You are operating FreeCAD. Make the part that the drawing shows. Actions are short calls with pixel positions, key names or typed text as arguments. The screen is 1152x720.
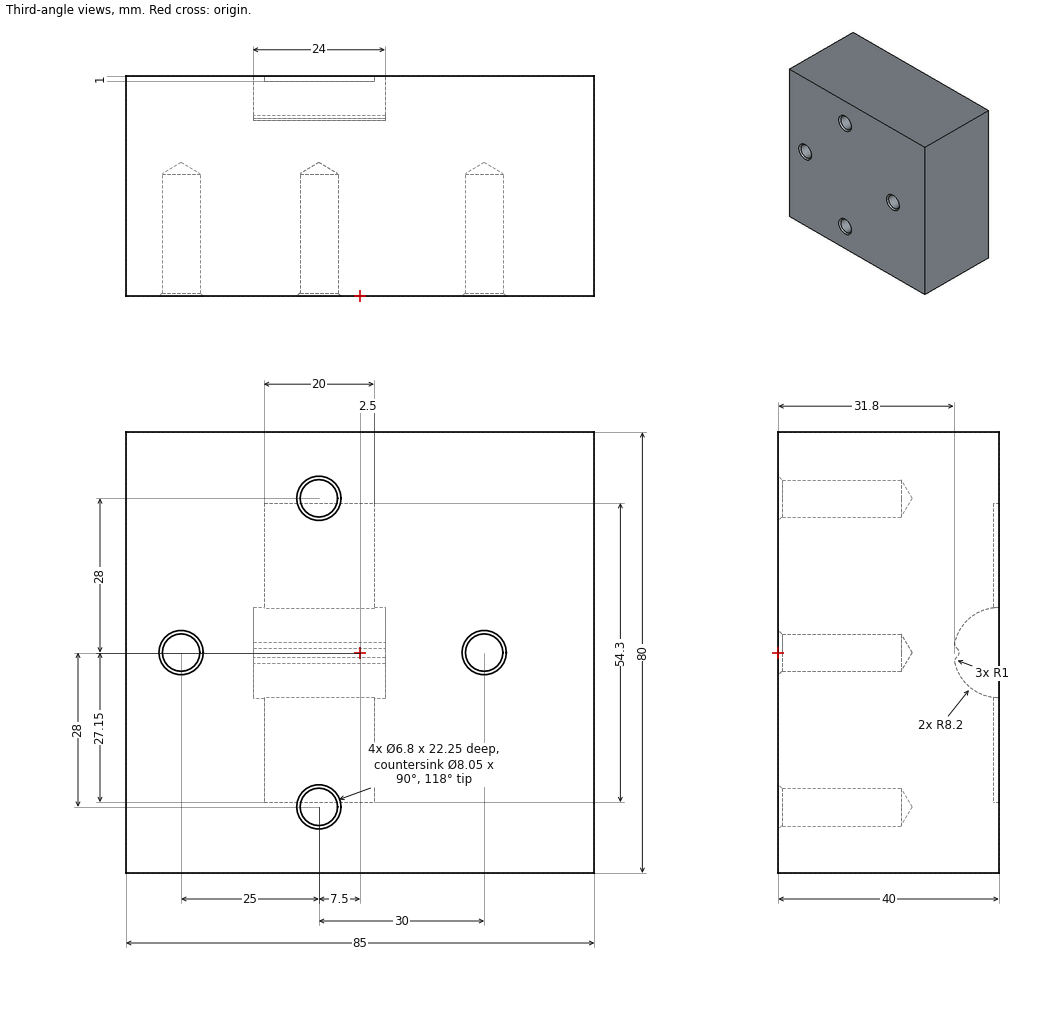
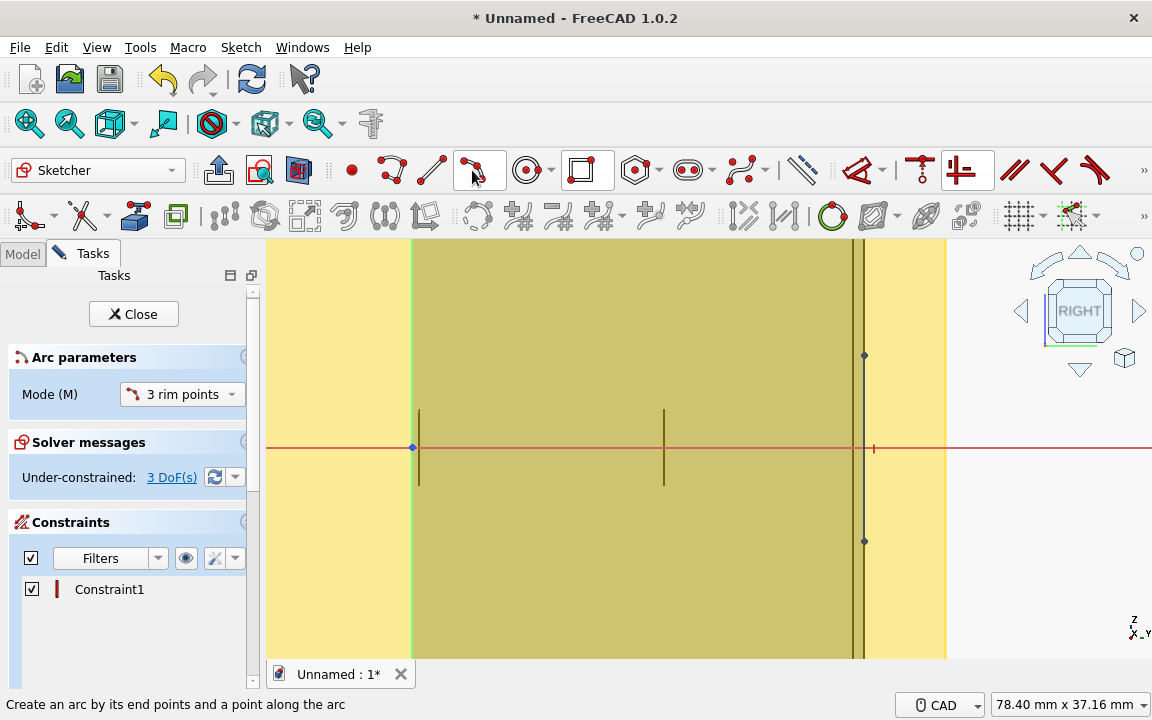
click(864, 542)
click(774, 469)
click(806, 520)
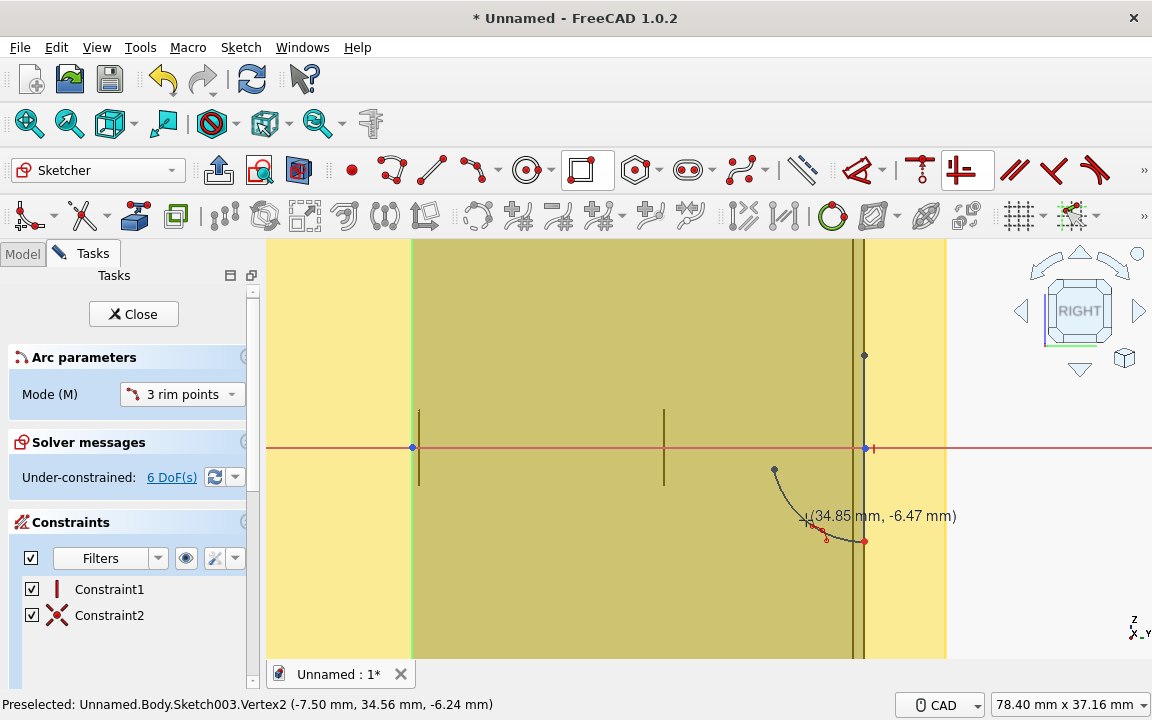
click(774, 470)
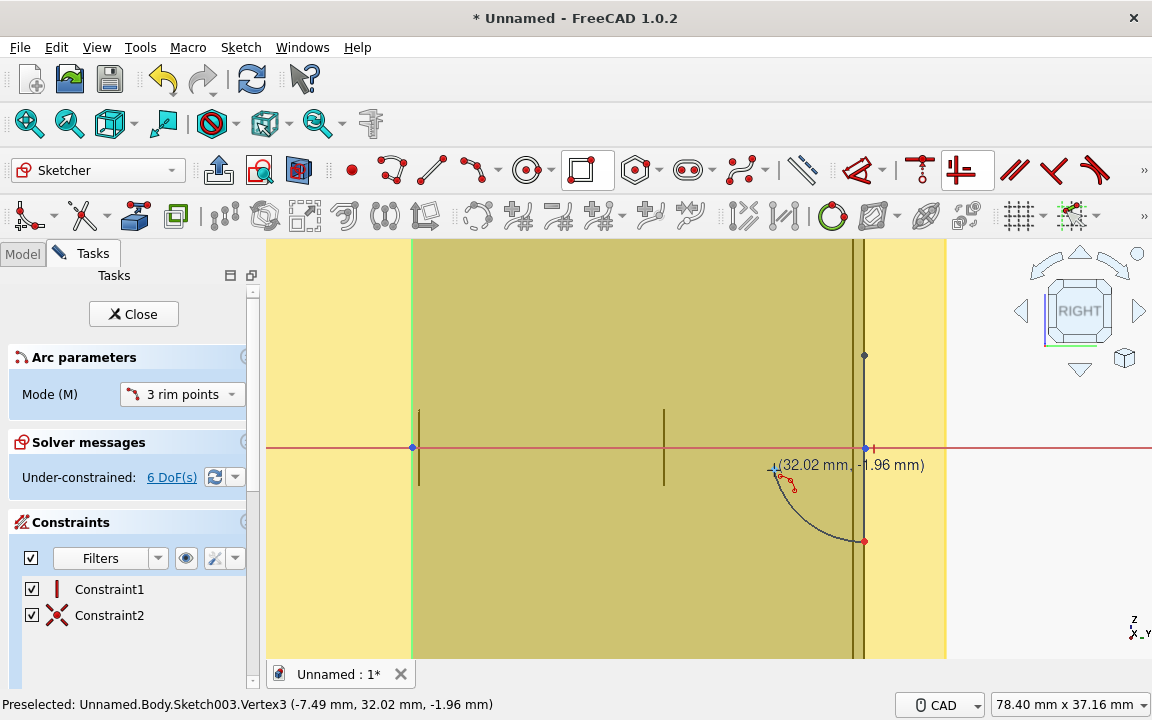
scroll(778, 457, up, 3)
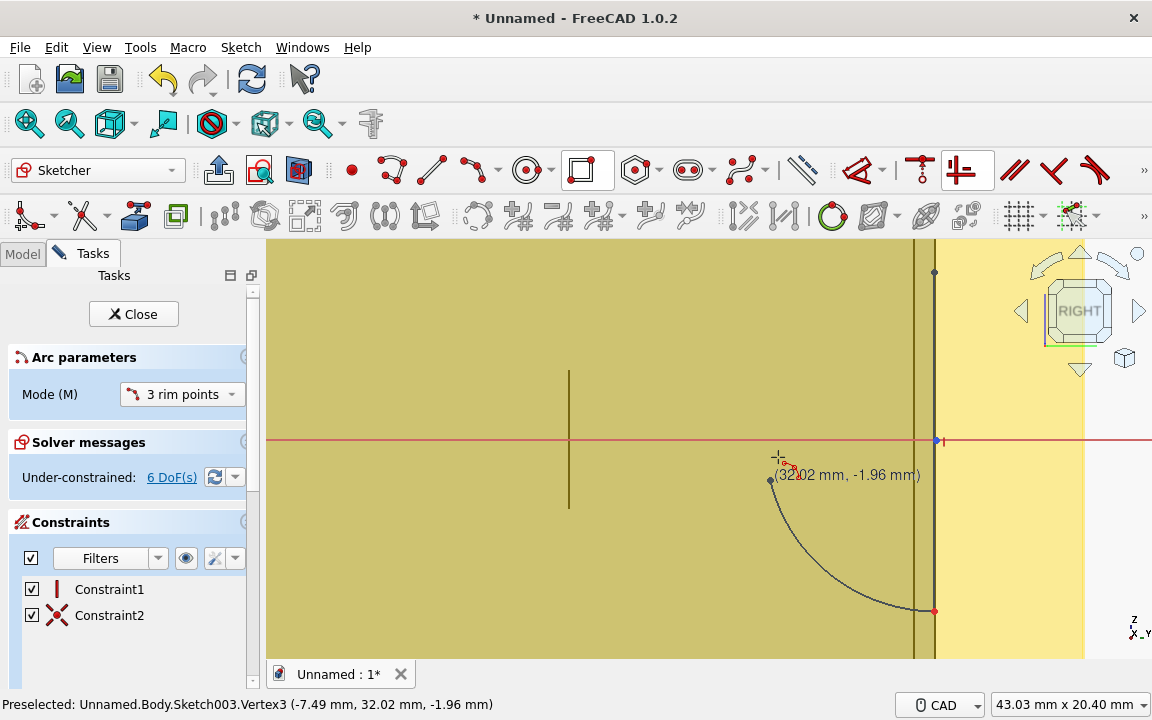
click(778, 456)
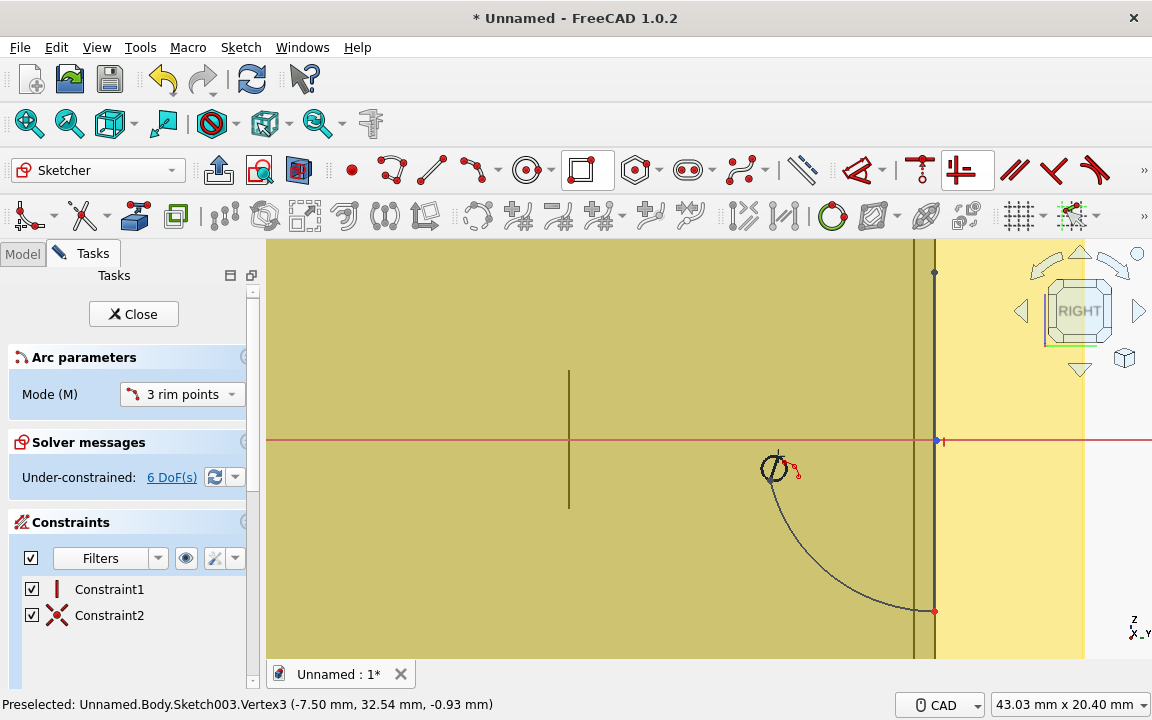
scroll(771, 466, up, 8)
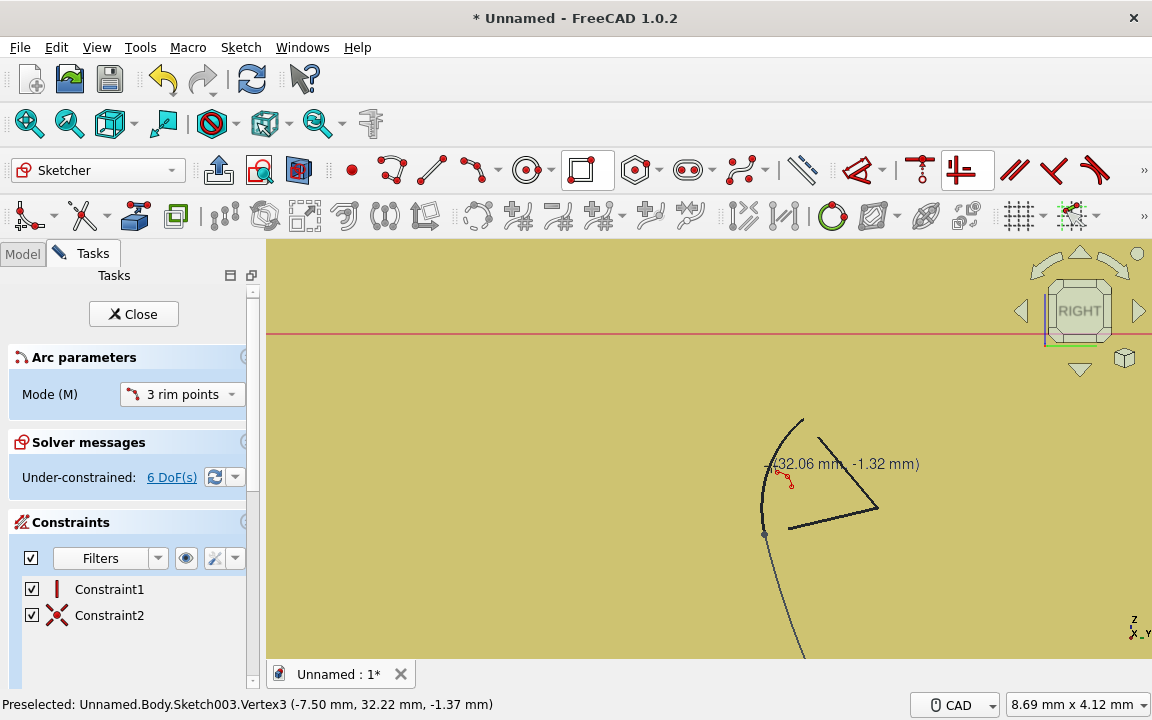
click(768, 463)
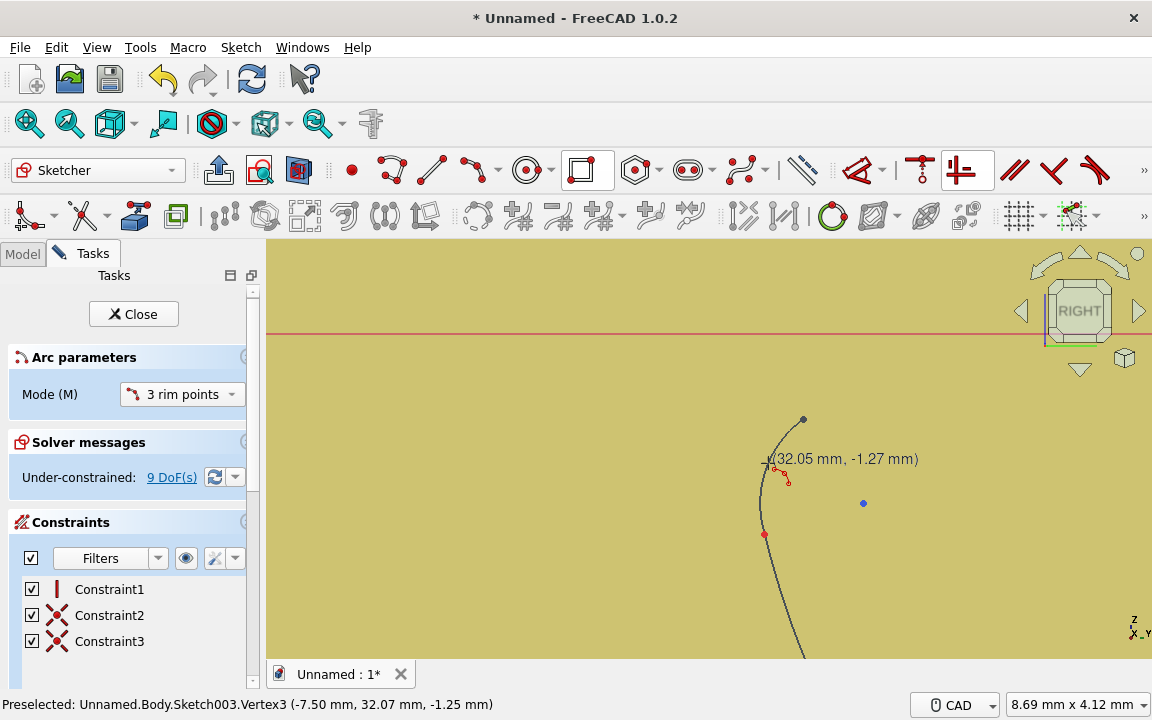
scroll(778, 463, down, 11)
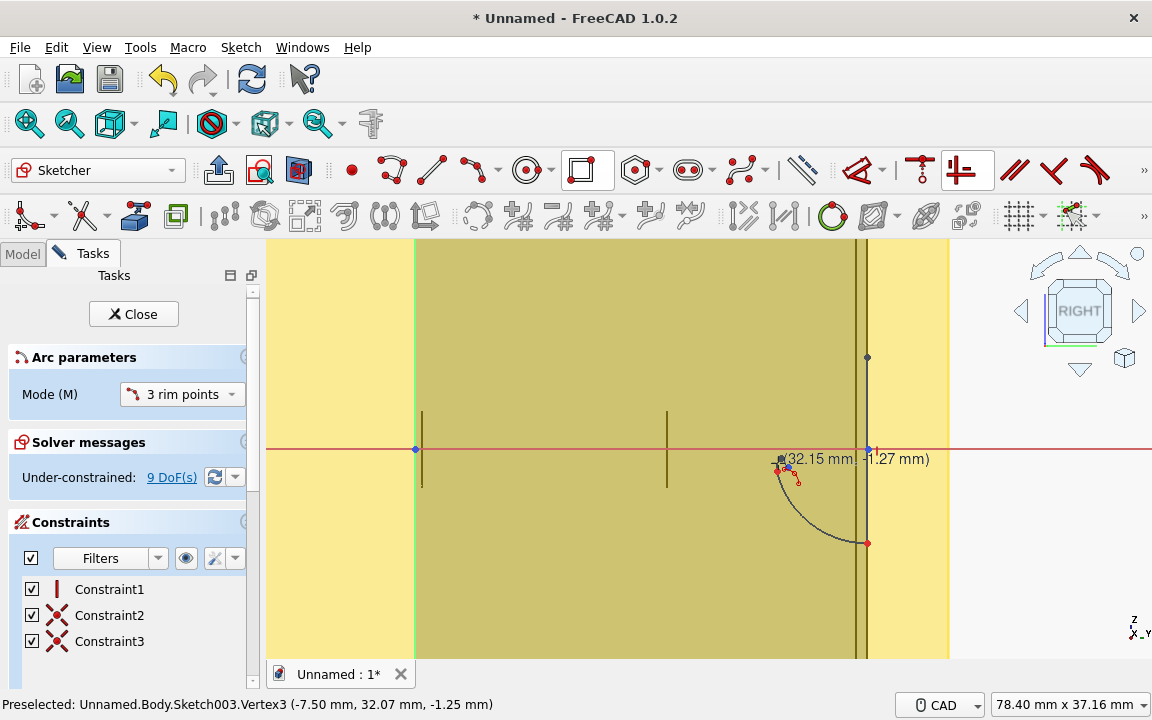
scroll(781, 458, up, 3)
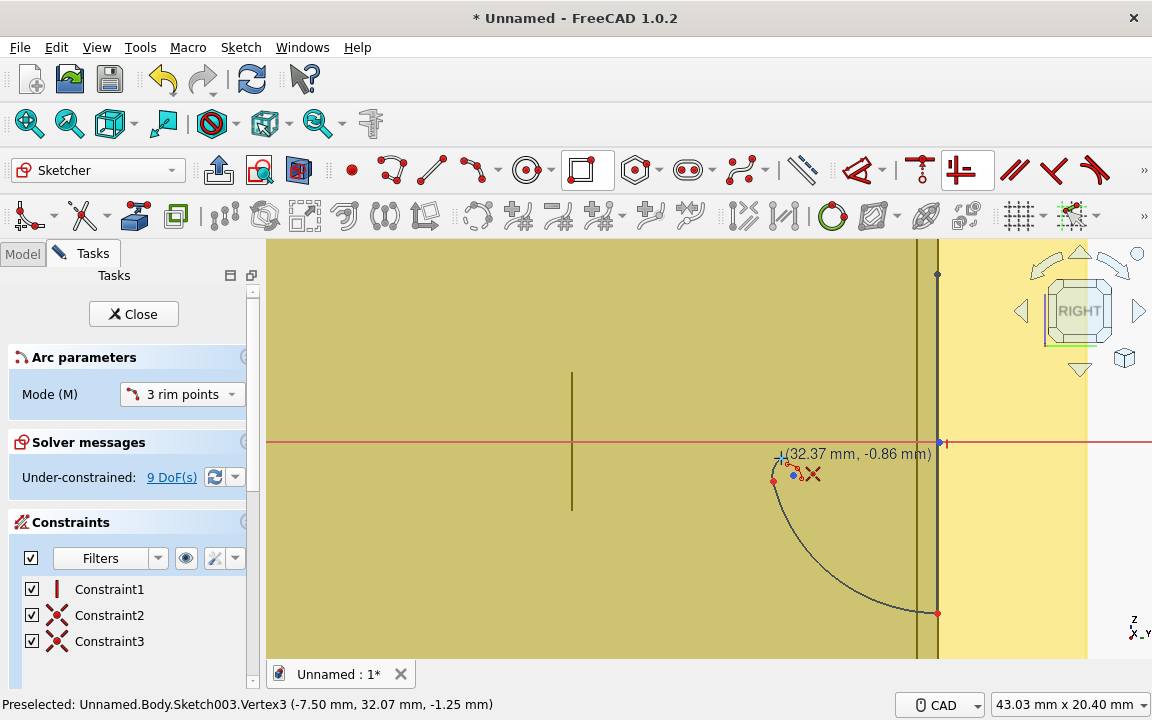
click(781, 459)
click(781, 425)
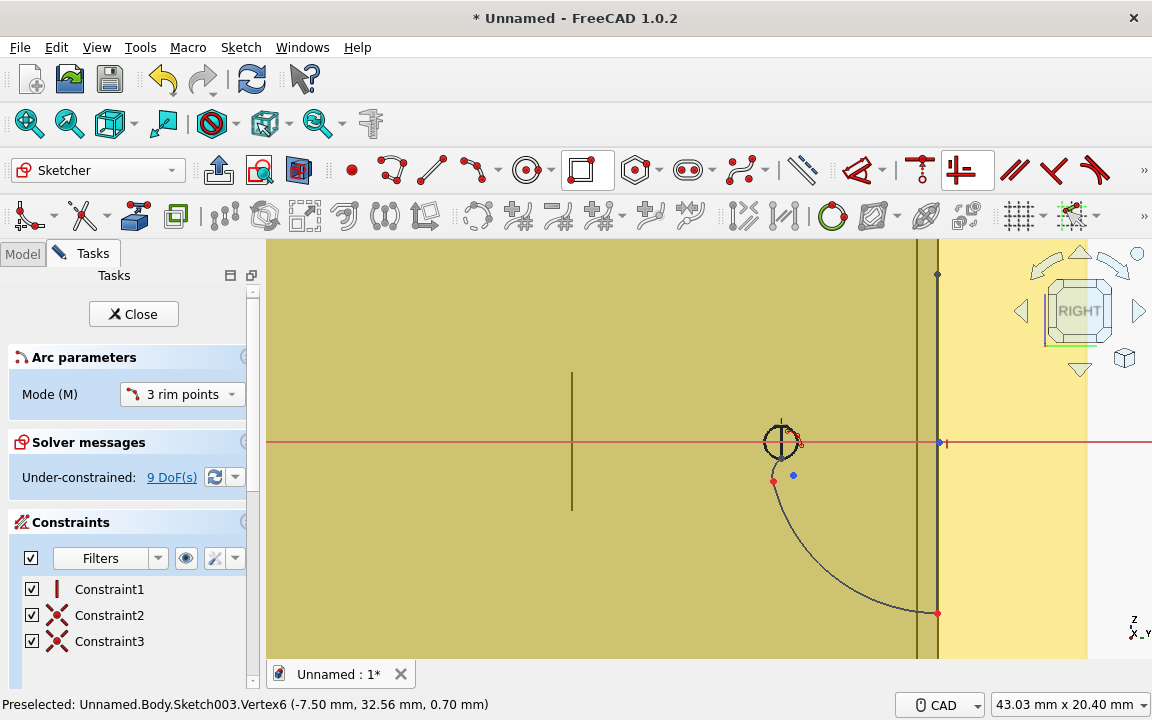
scroll(788, 449, up, 5)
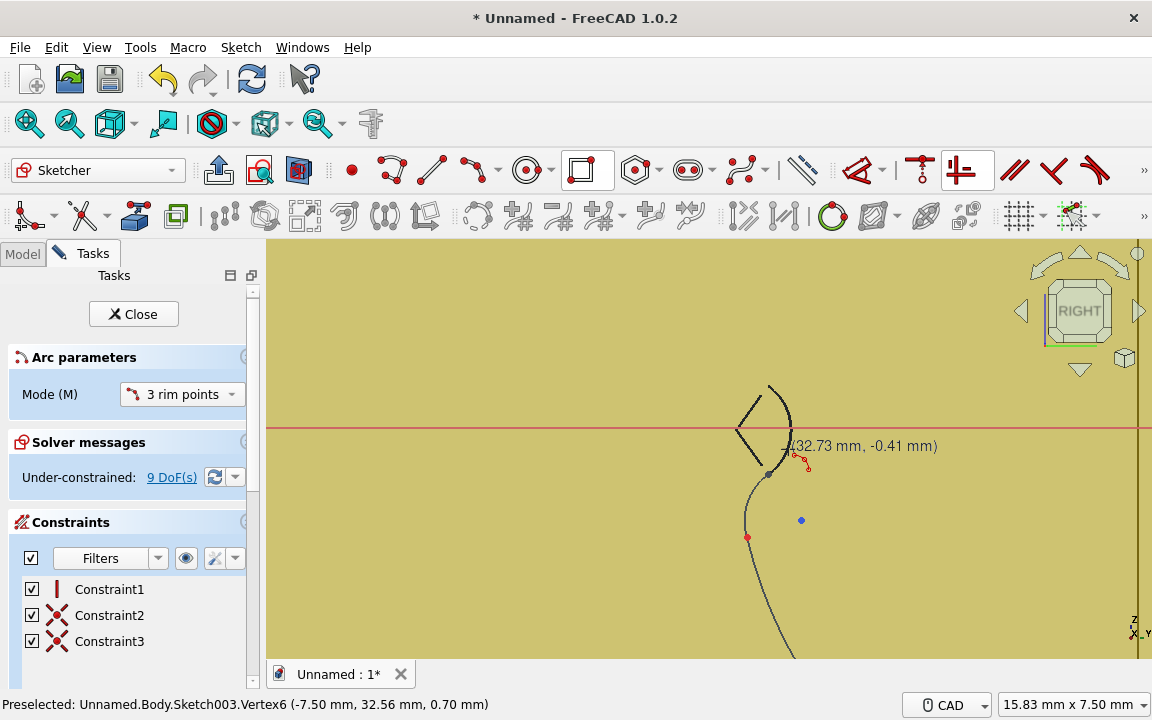
click(787, 449)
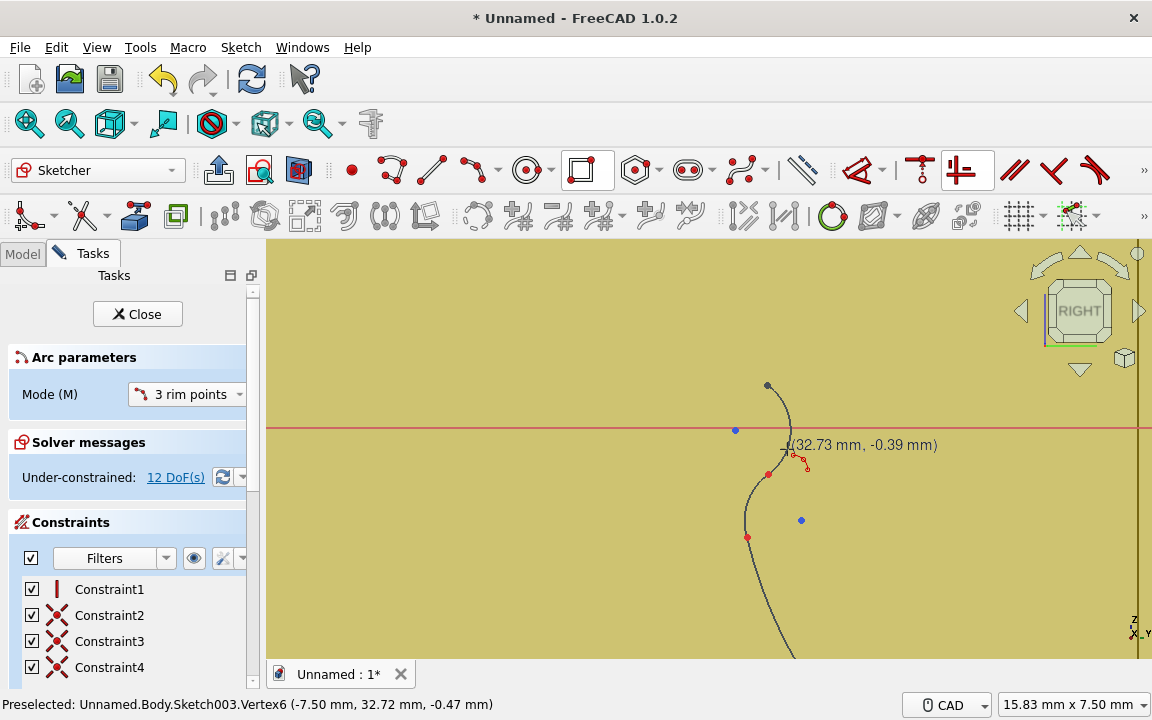
click(768, 386)